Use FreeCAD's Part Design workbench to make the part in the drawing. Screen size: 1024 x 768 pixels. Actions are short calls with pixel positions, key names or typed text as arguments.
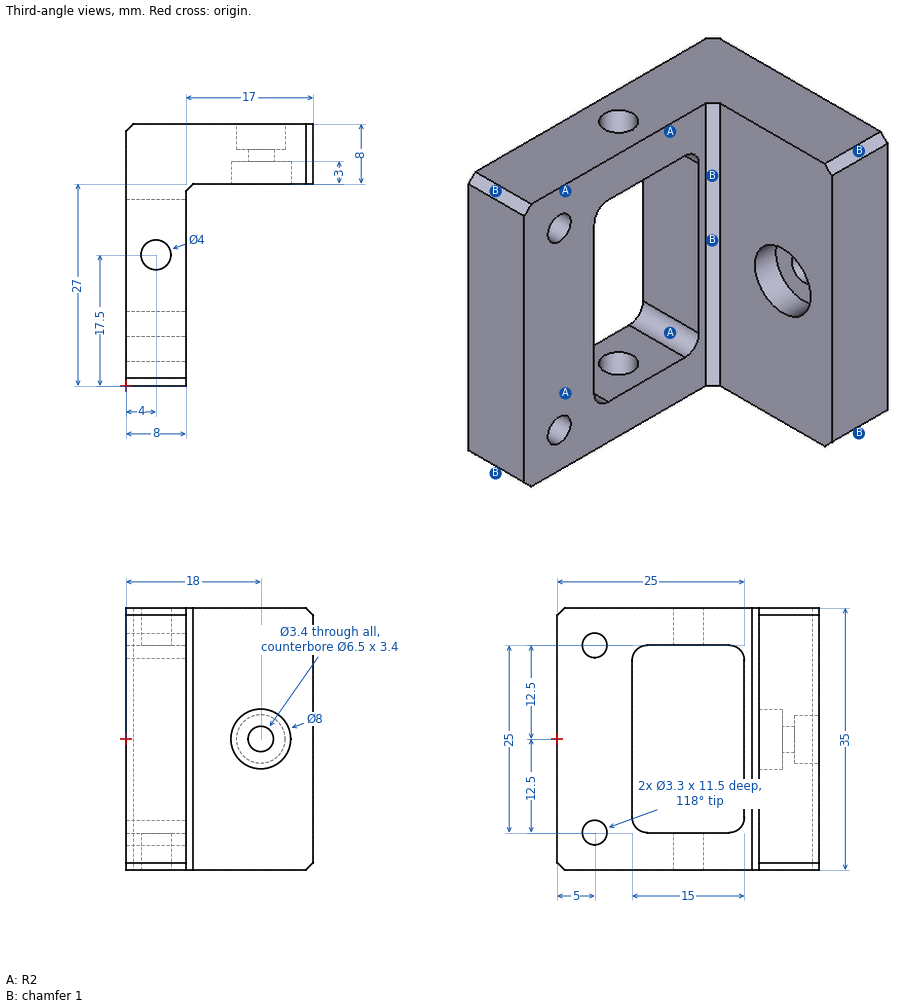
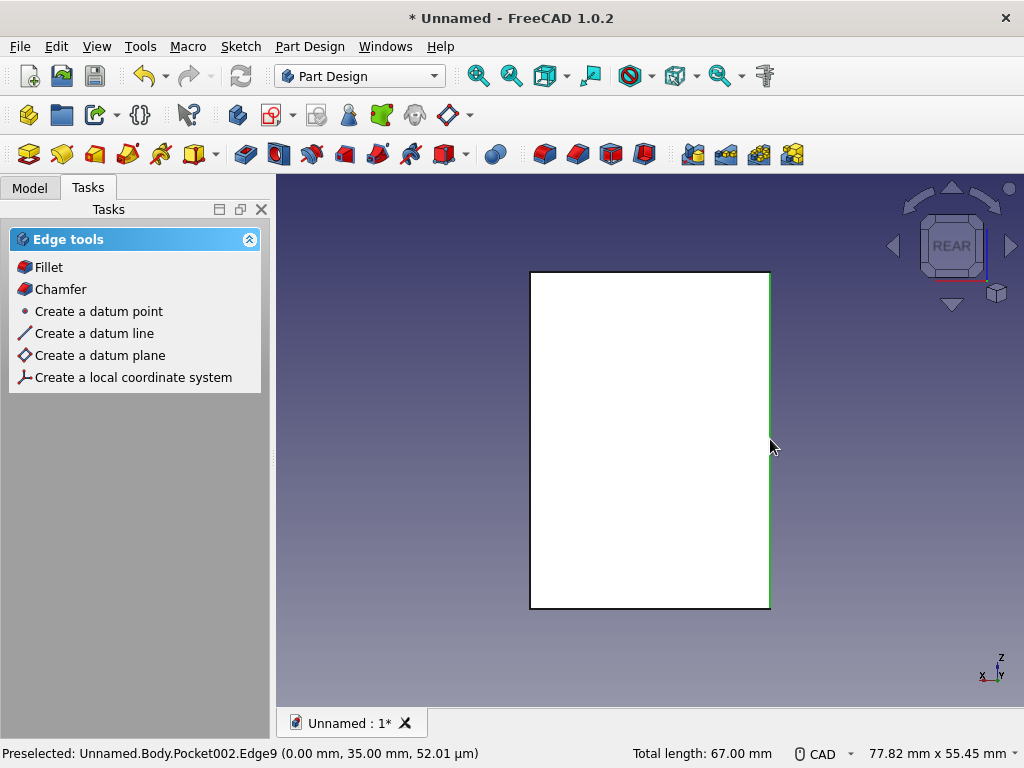
key(6)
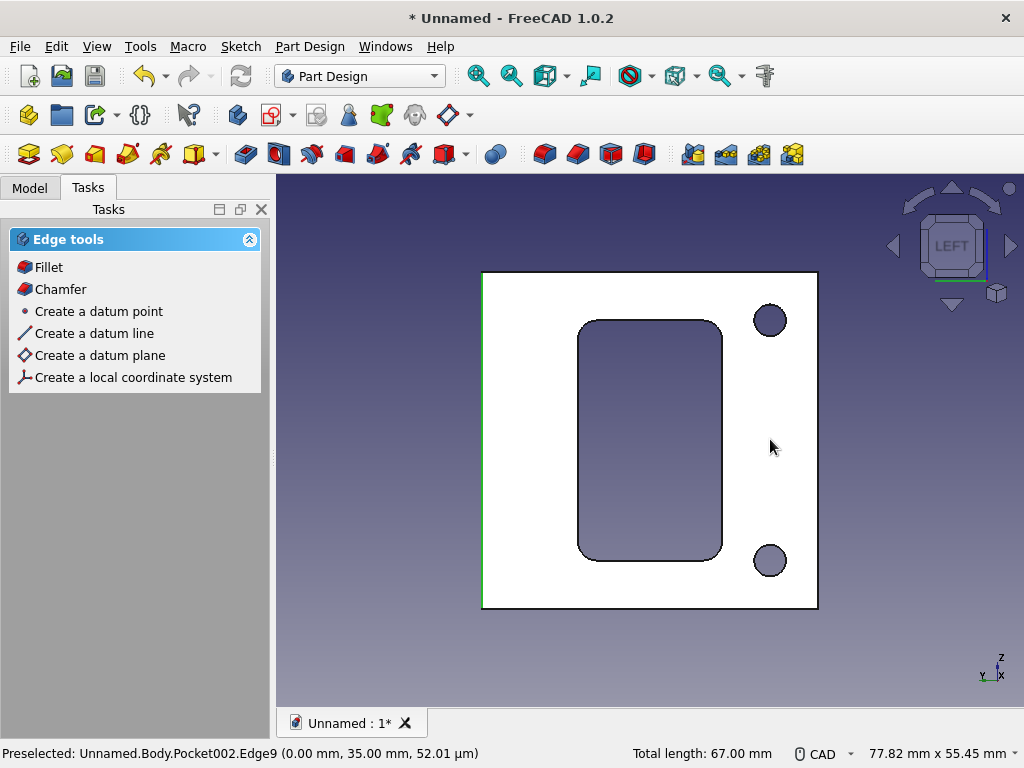
key(v)
key(3)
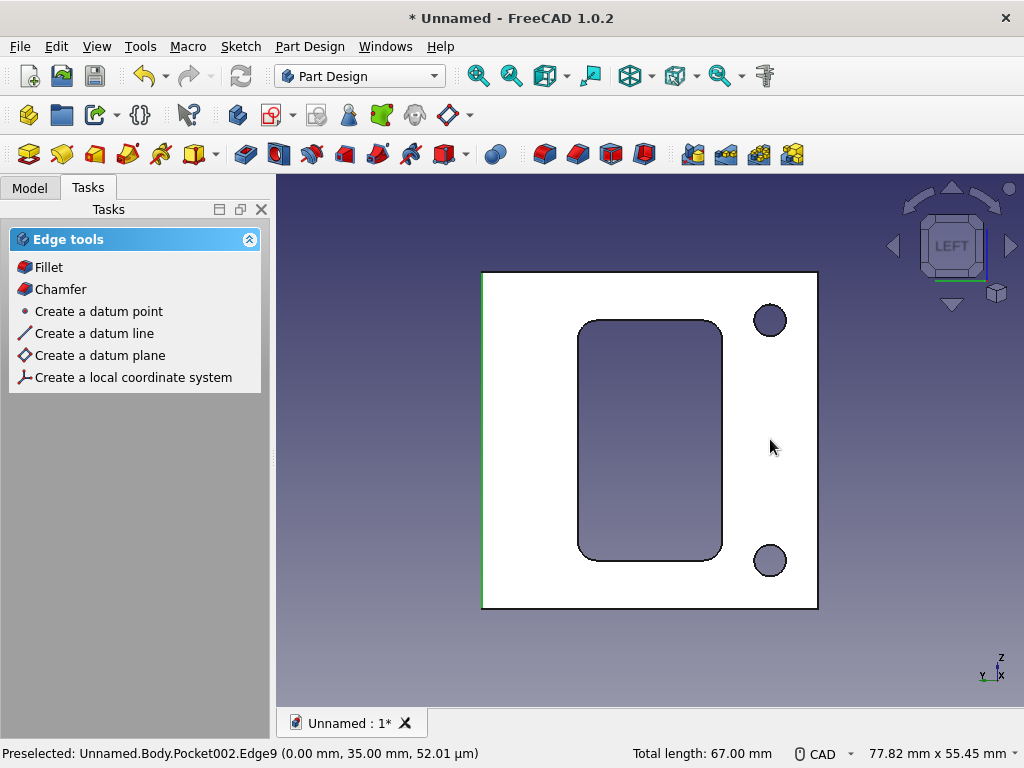
key(0)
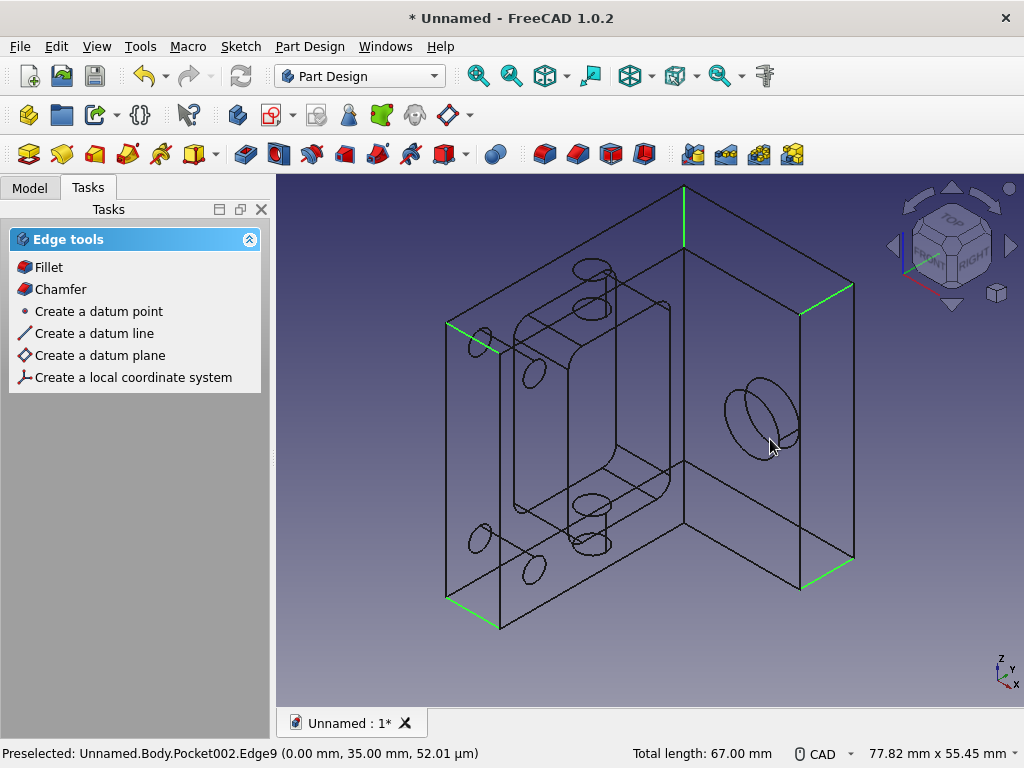
click(684, 385, ctrl)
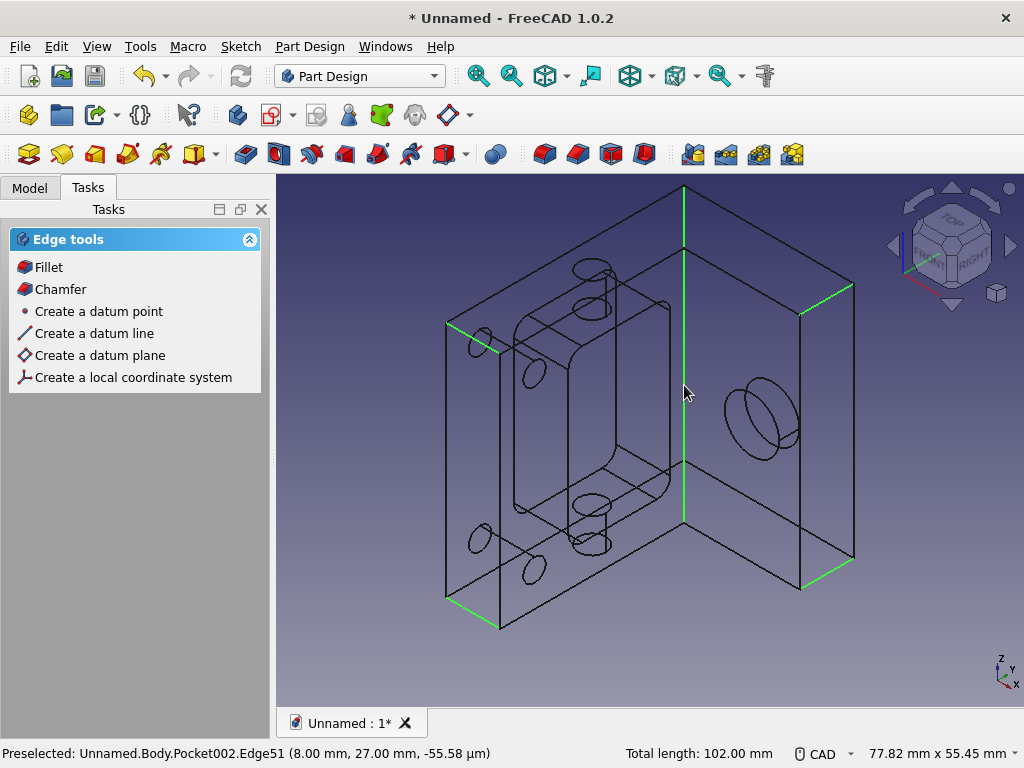
key(v)
key(1)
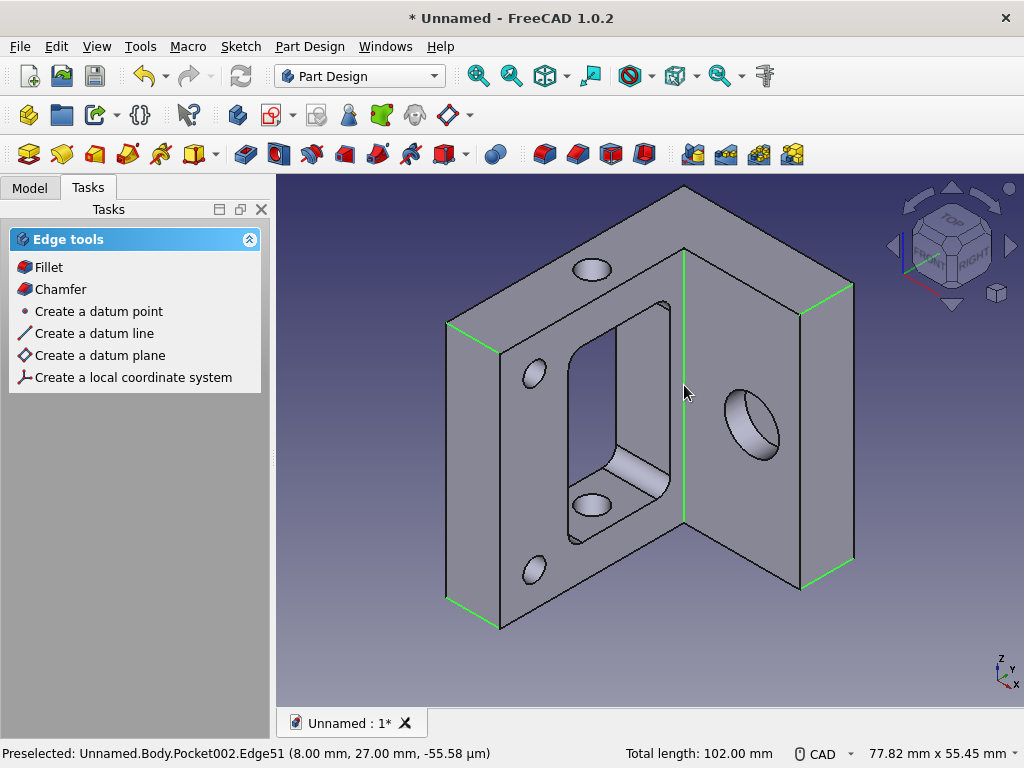
click(578, 154)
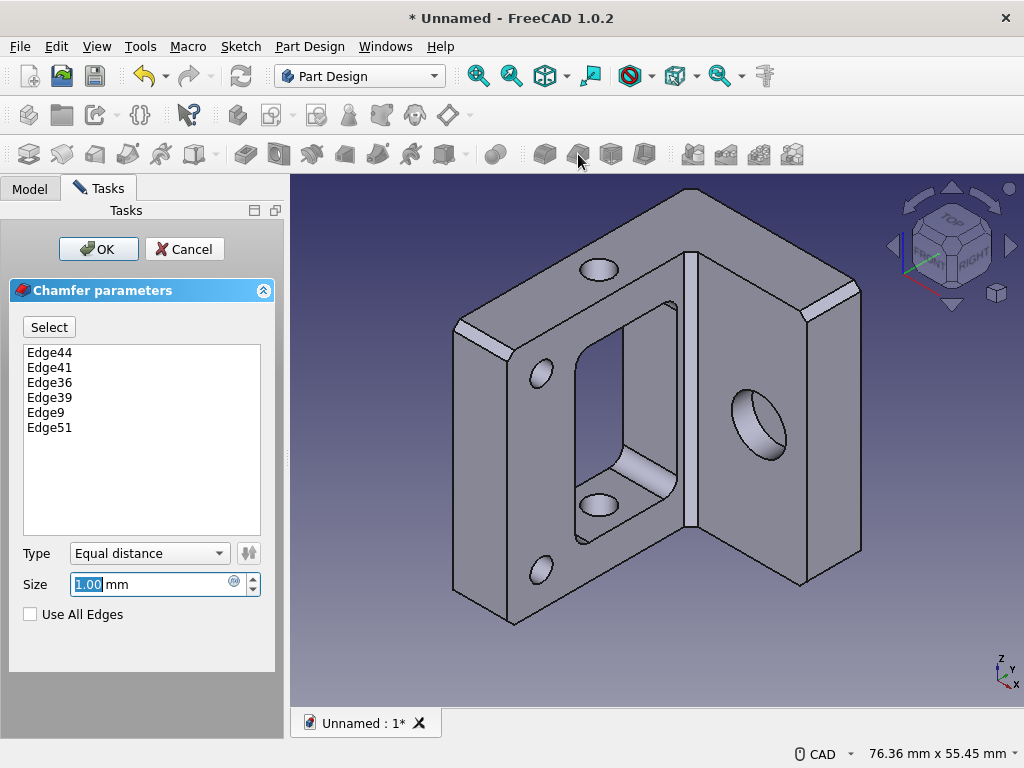
text(1)
key(Tab)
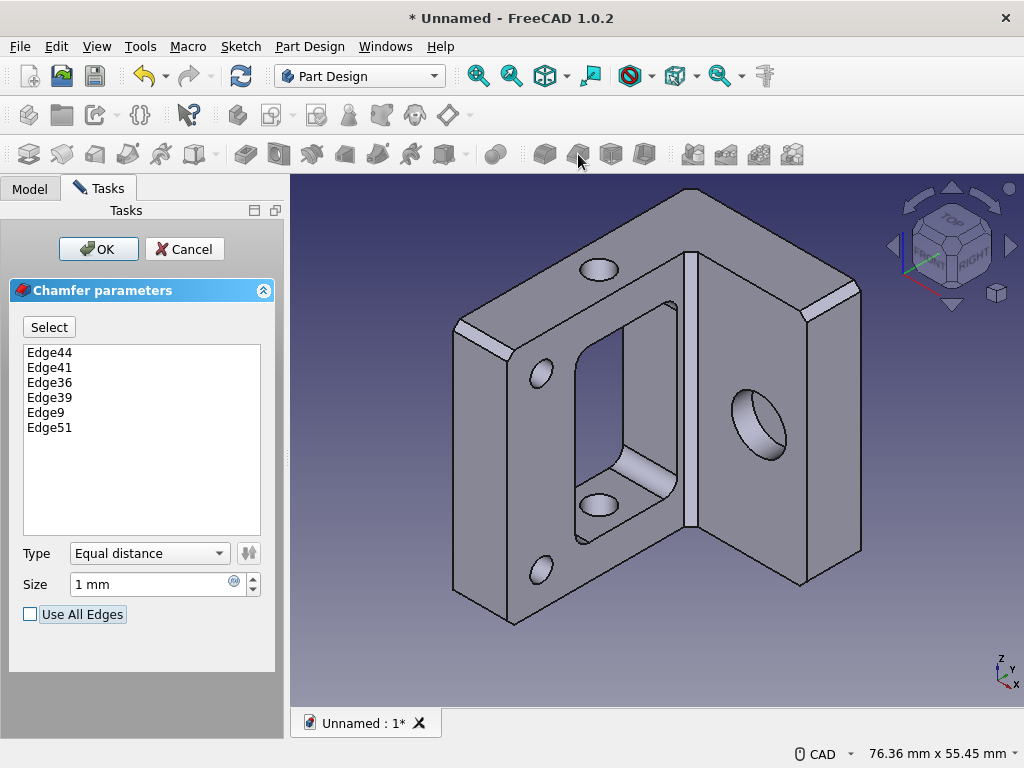
click(99, 249)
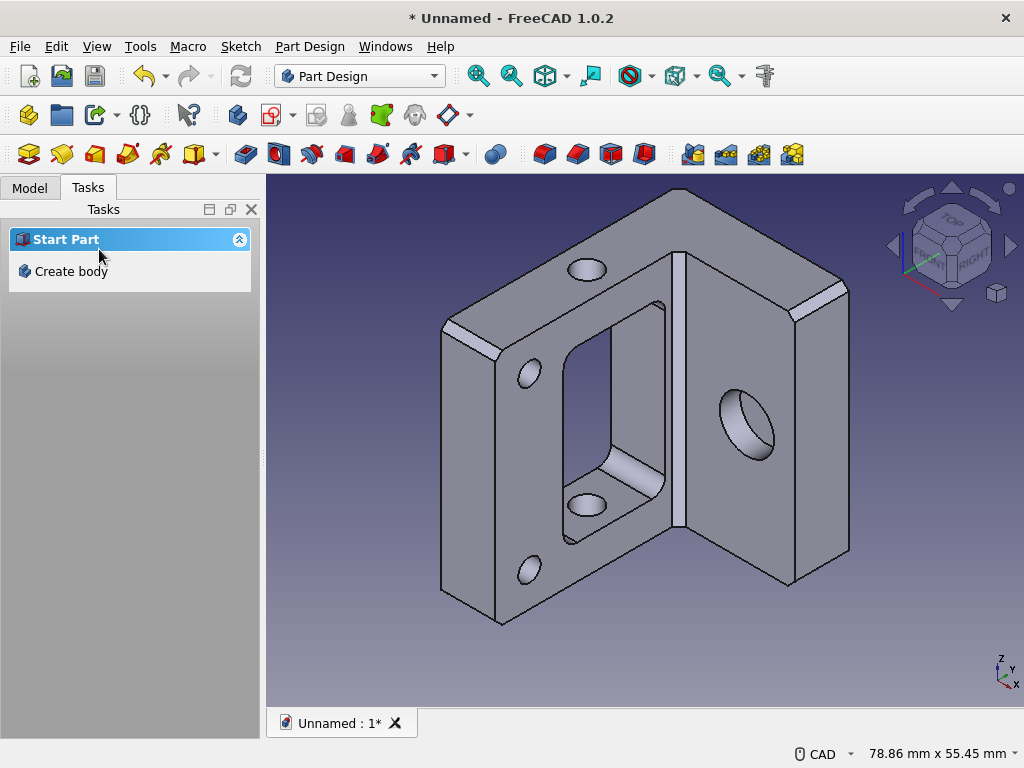
key(4)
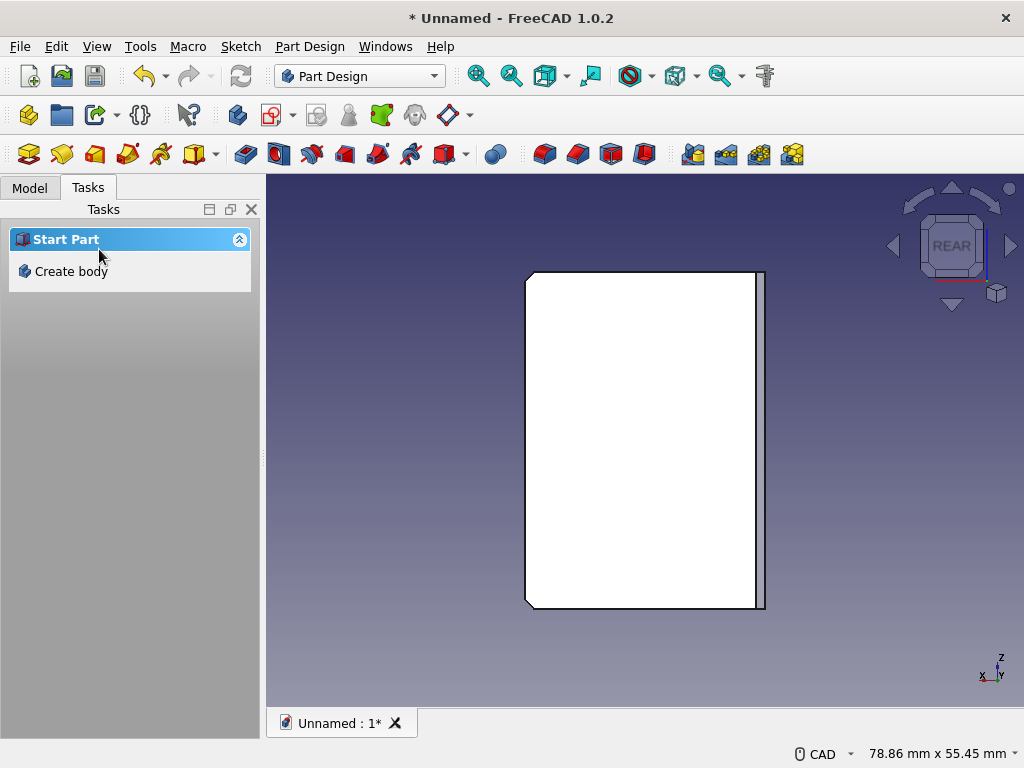
click(640, 391)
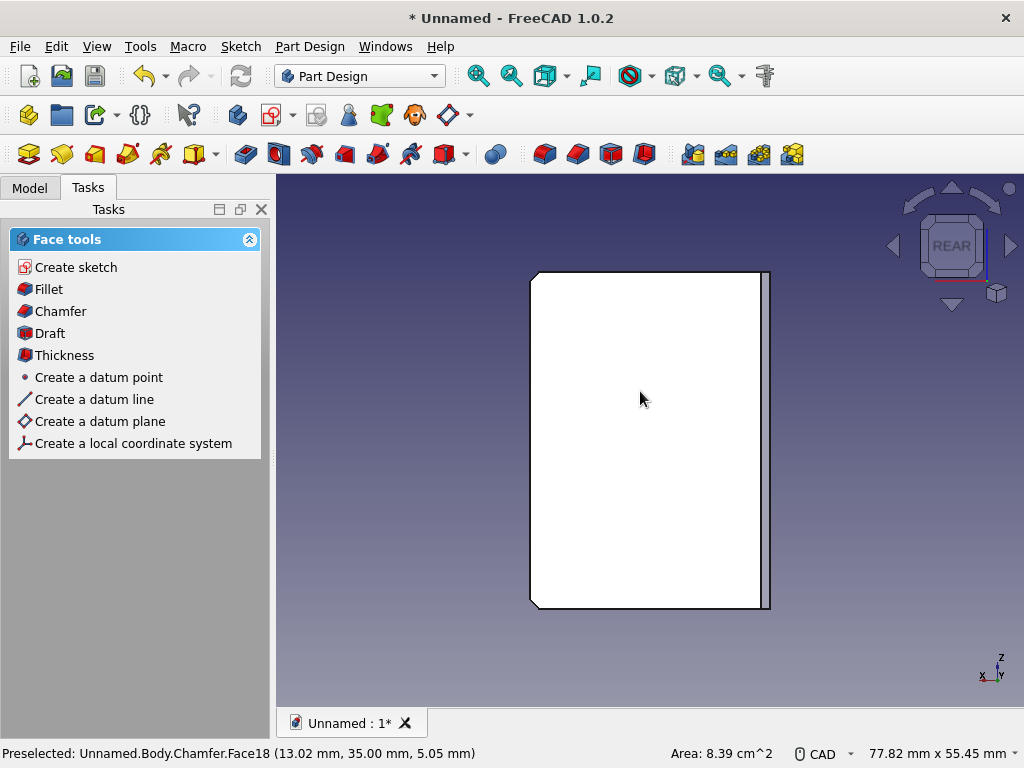
click(270, 116)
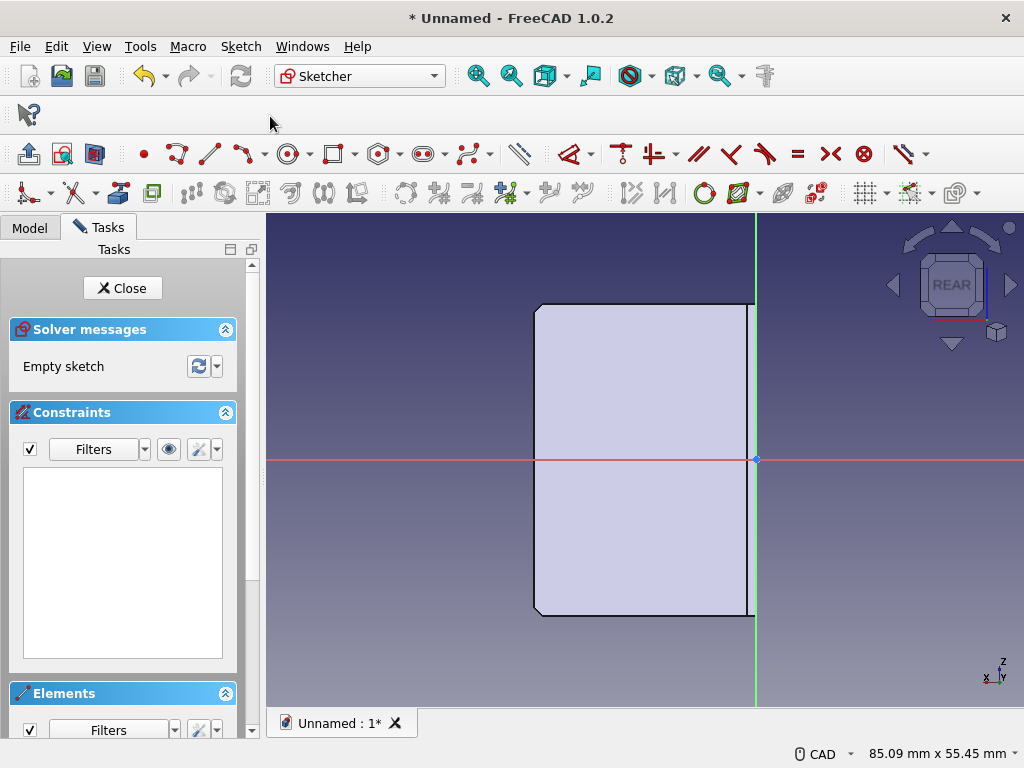
scroll(598, 460, up, 12)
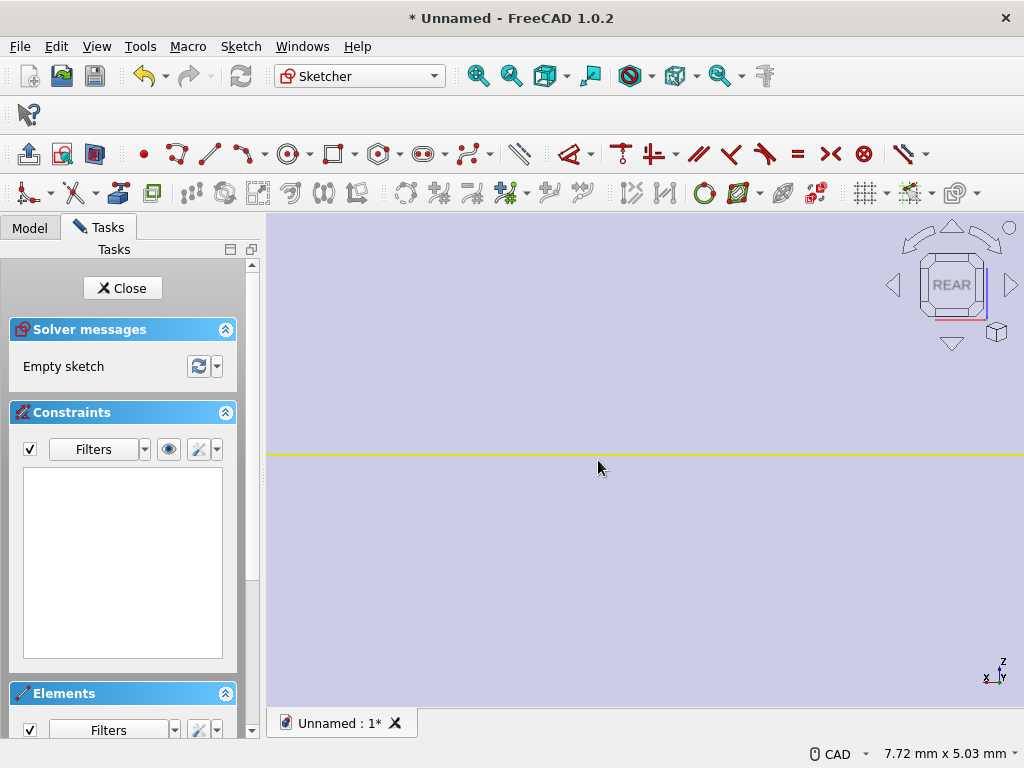
click(288, 154)